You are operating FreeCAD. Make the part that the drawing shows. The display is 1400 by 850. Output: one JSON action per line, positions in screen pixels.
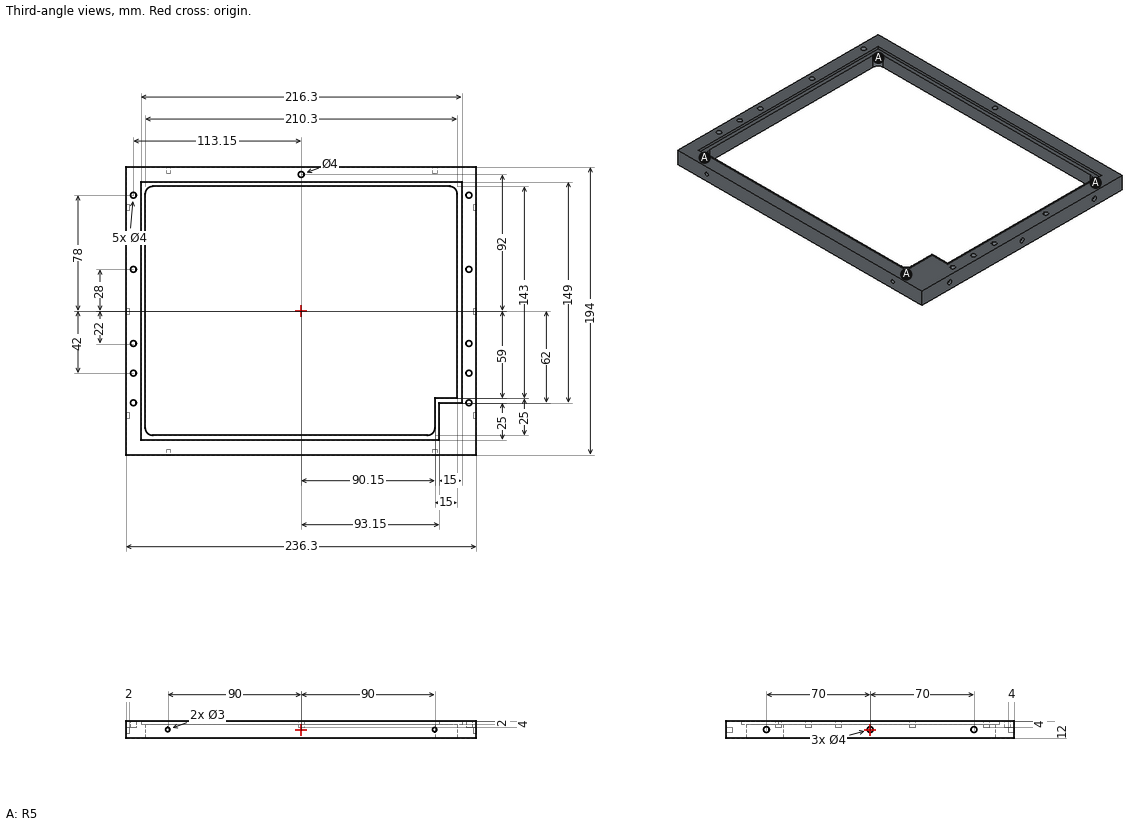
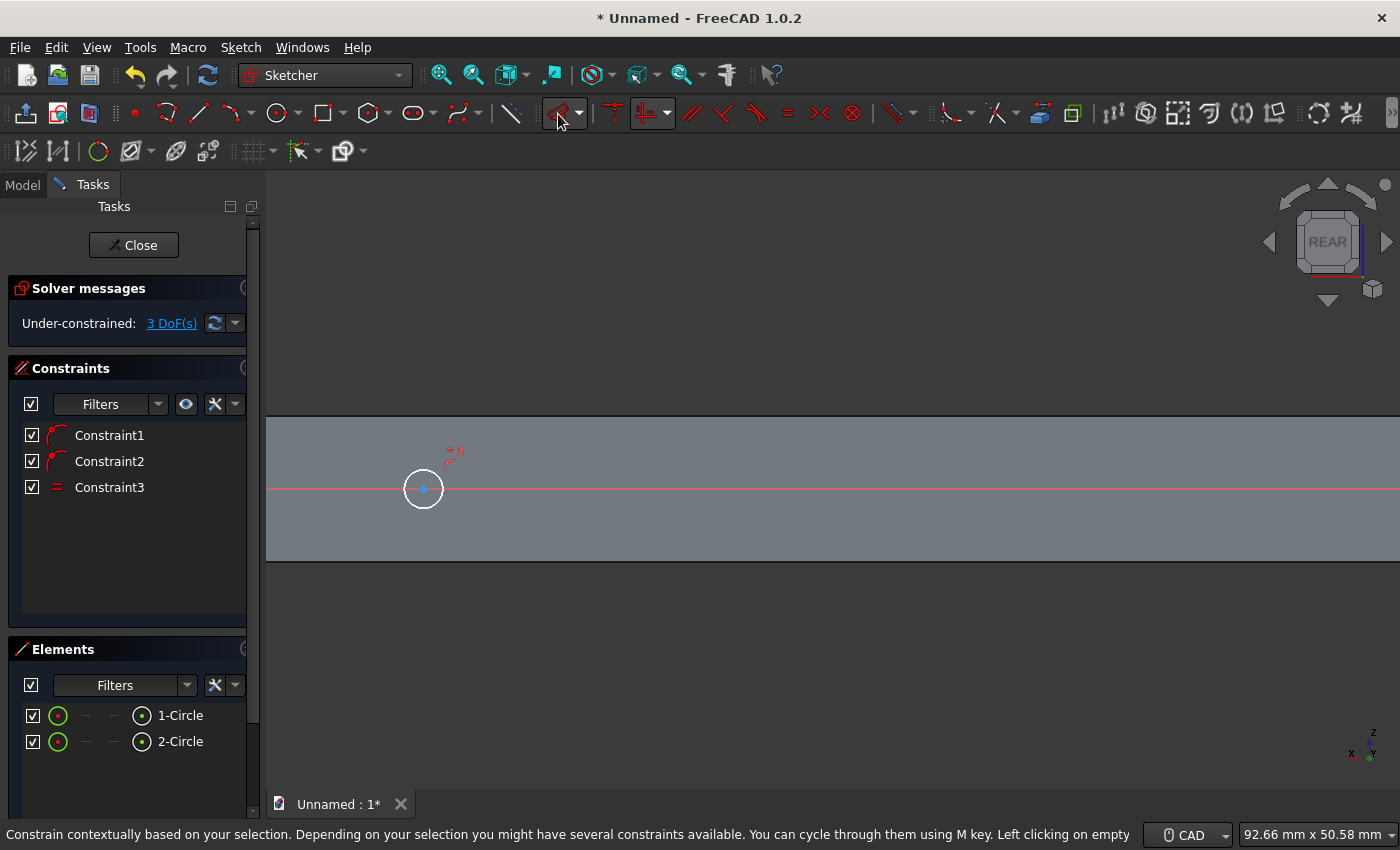
{"action": "scroll", "coordinate": [437, 475], "scroll_direction": "down", "scroll_amount": 6}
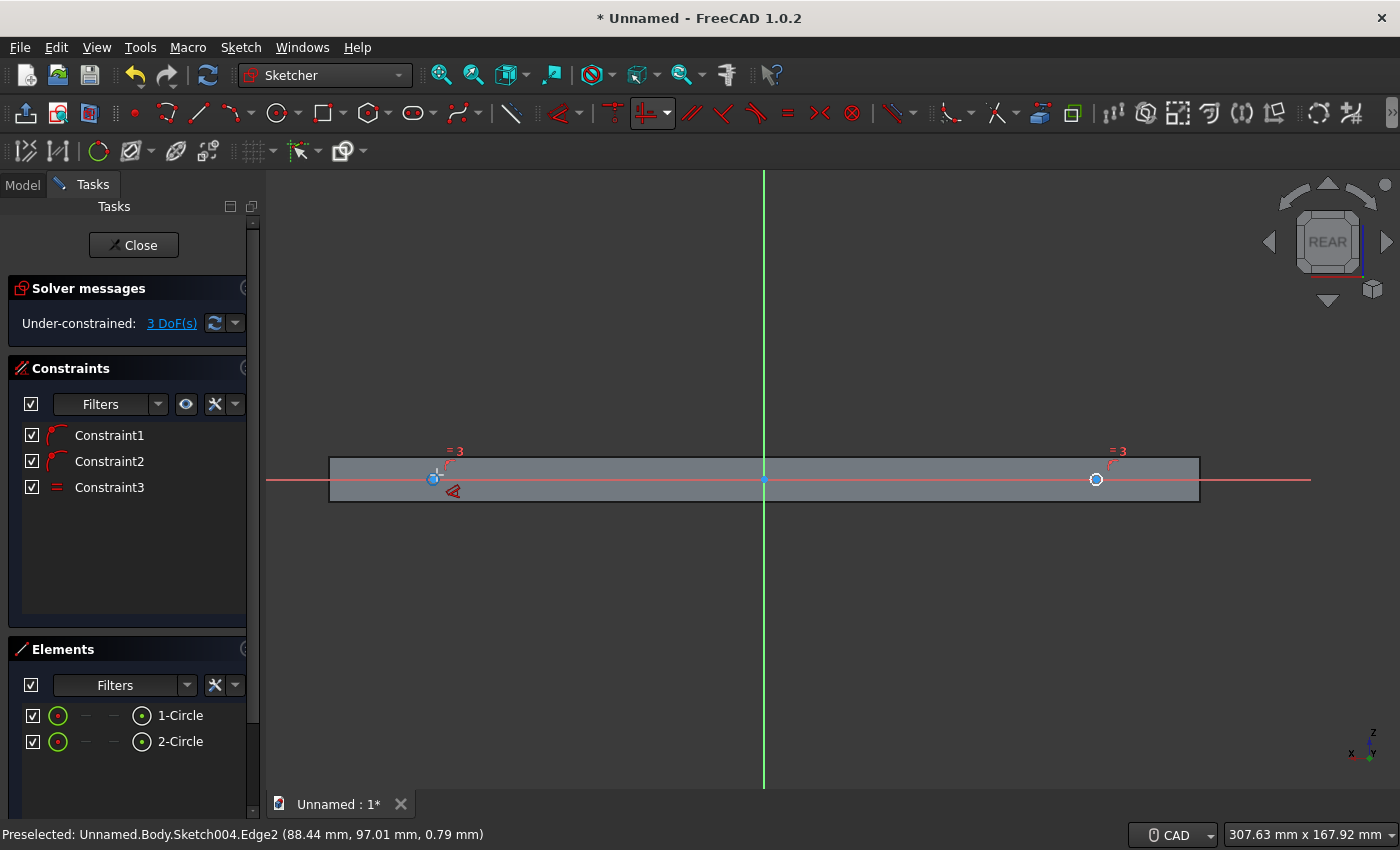
{"action": "scroll", "coordinate": [1100, 475], "scroll_direction": "up", "scroll_amount": 7}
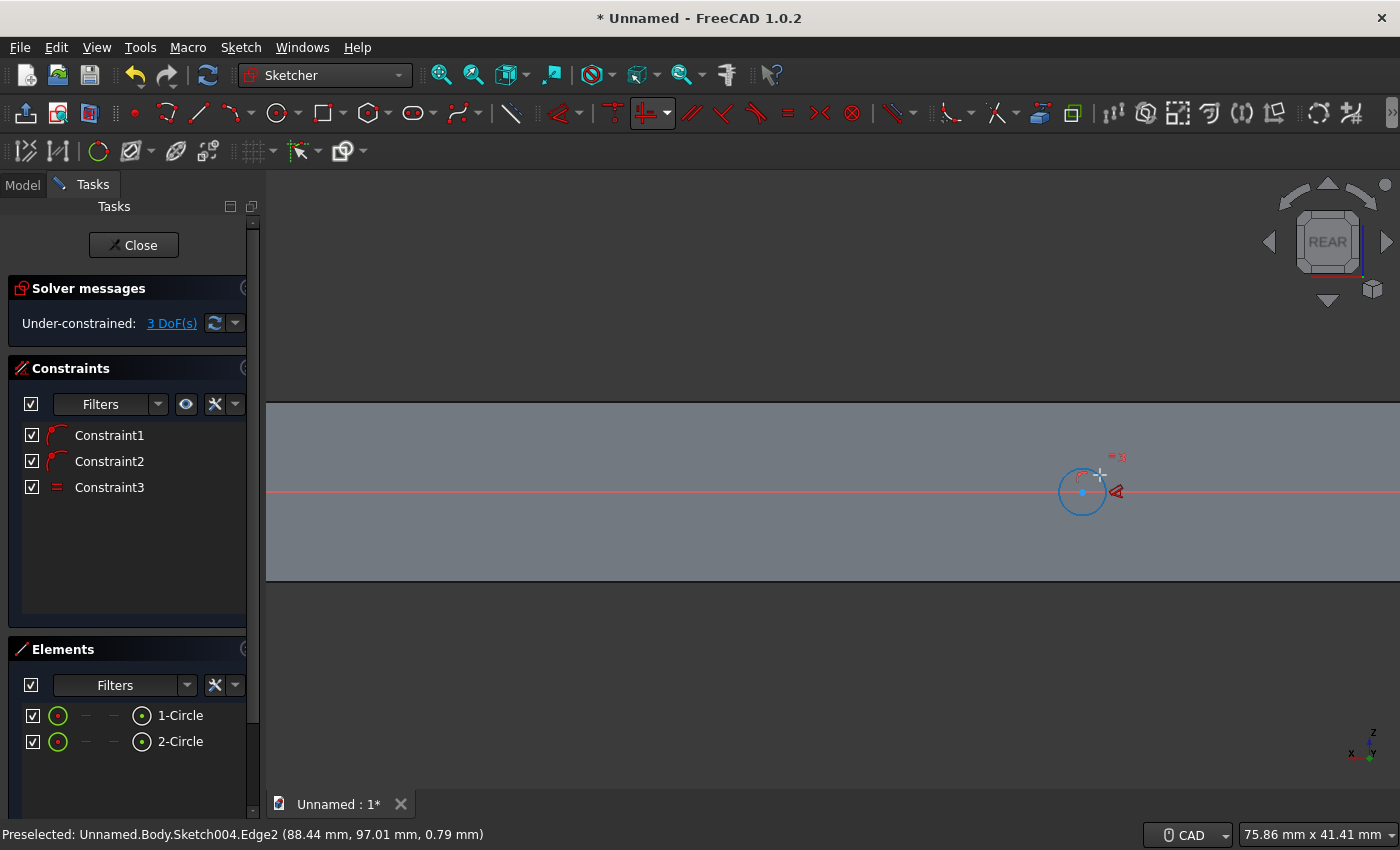
{"action": "left_click", "coordinate": [1099, 475]}
{"action": "left_click", "coordinate": [1121, 452]}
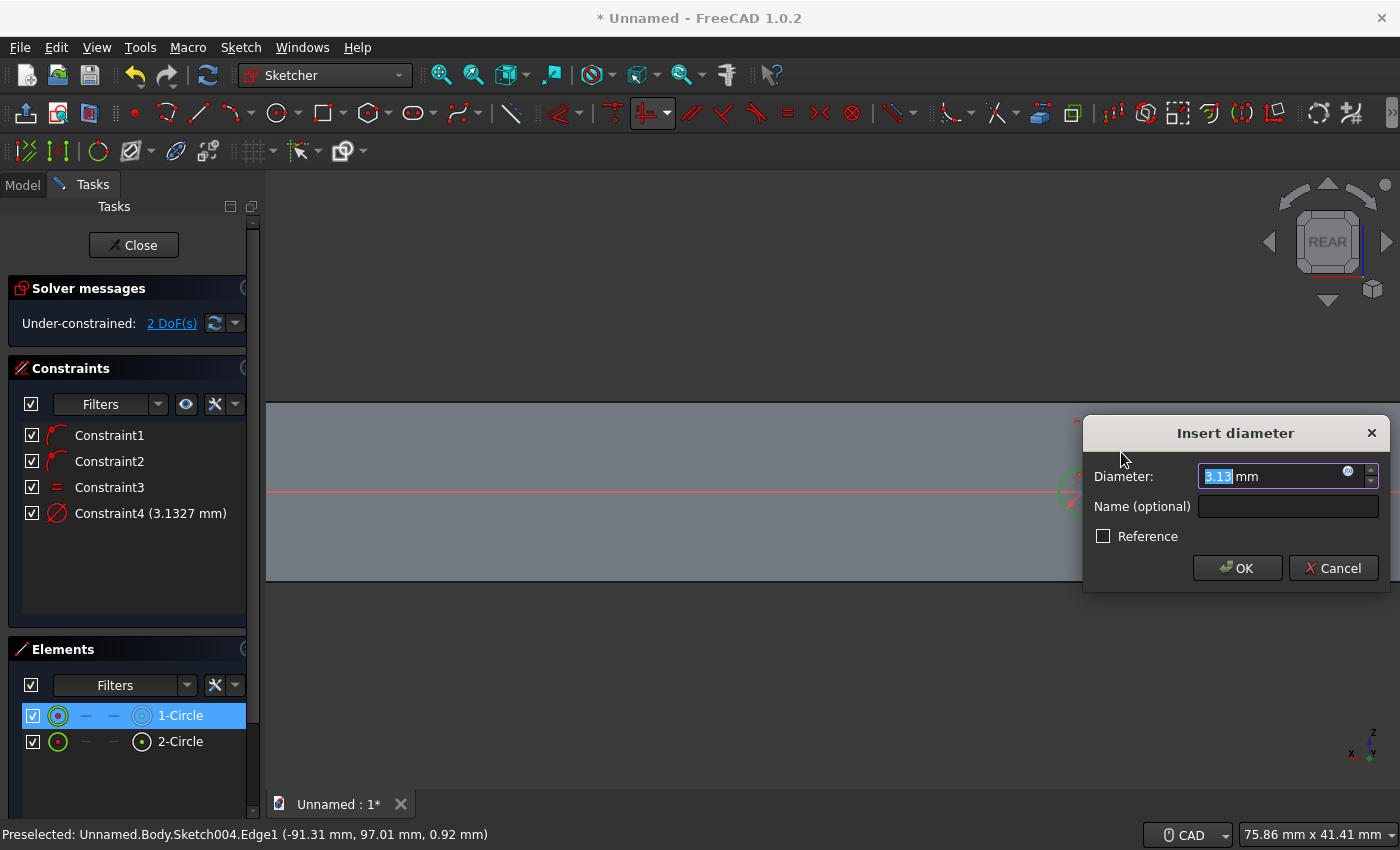
{"action": "type", "text": "3"}
{"action": "key", "text": "Return"}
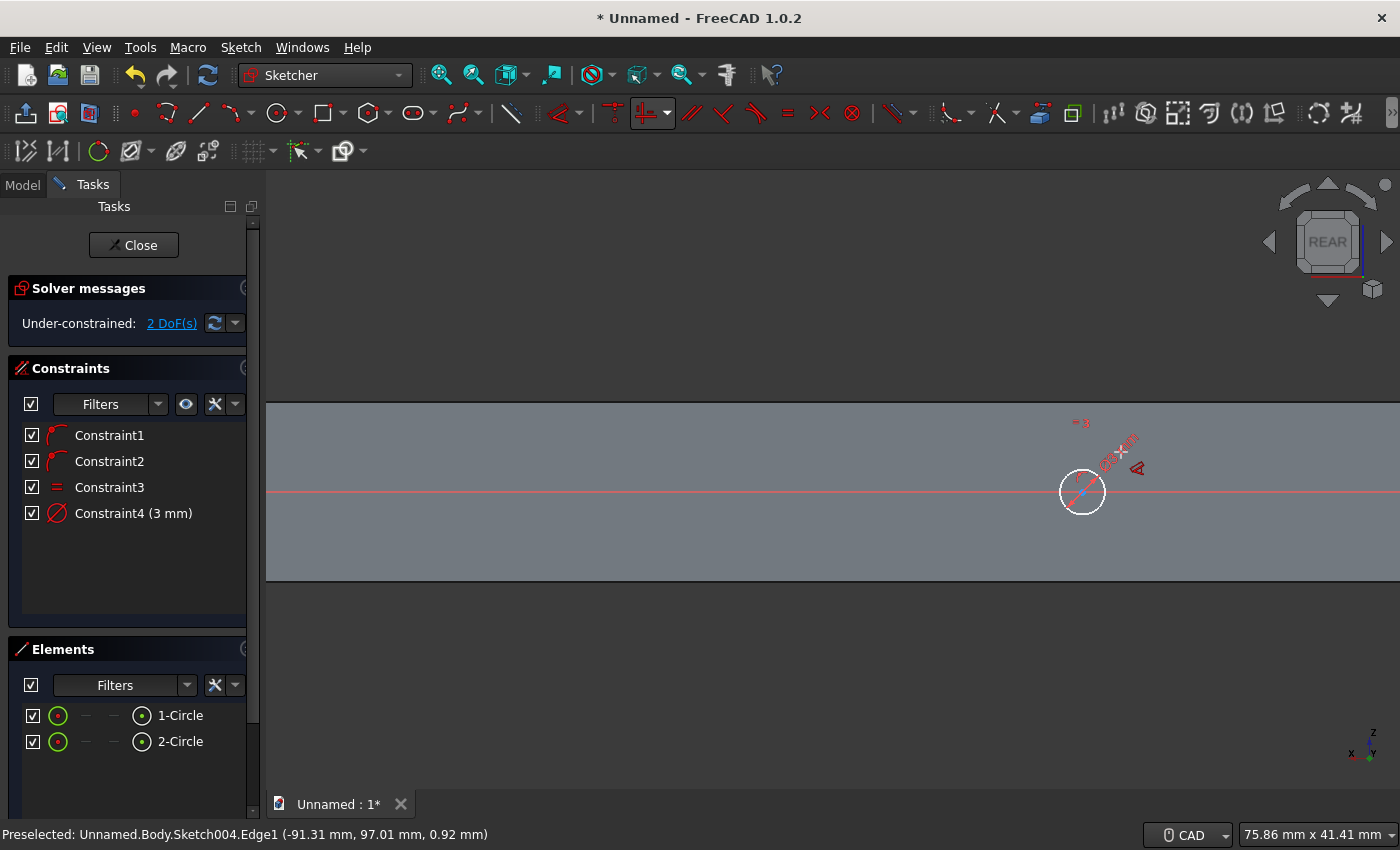
{"action": "scroll", "coordinate": [1101, 475], "scroll_direction": "down", "scroll_amount": 7}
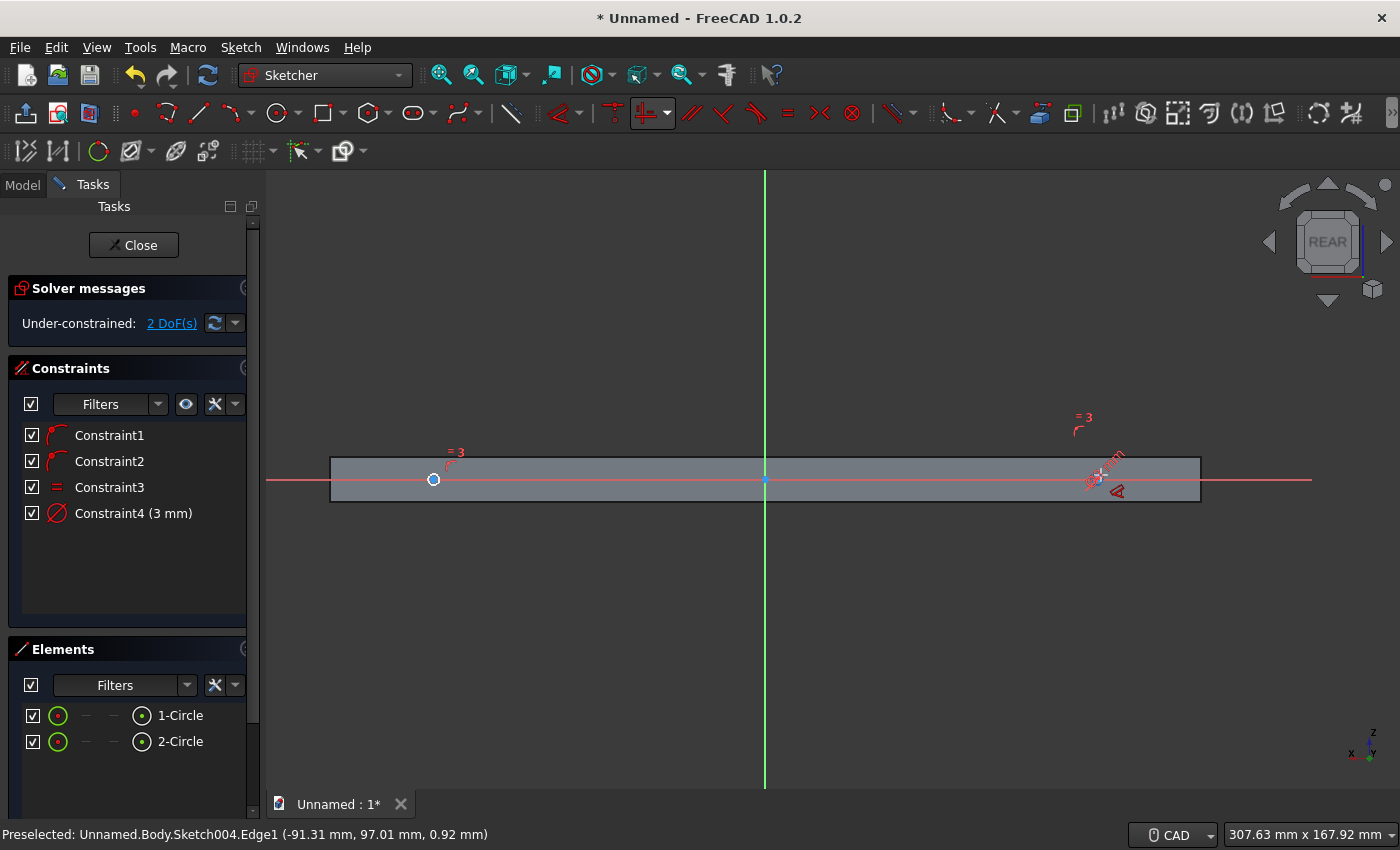
{"action": "left_click", "coordinate": [1097, 480]}
{"action": "left_click", "coordinate": [931, 514]}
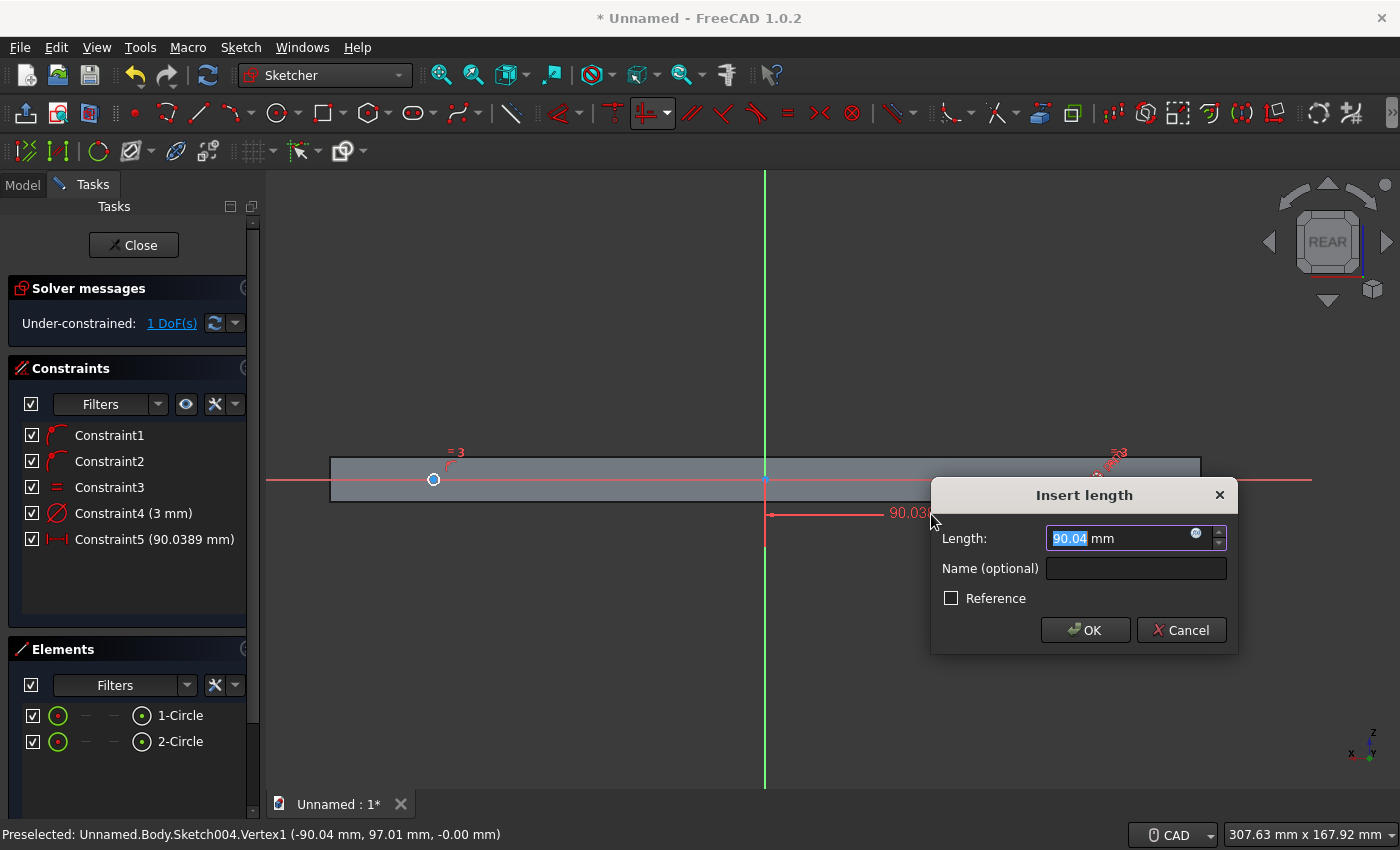
{"action": "type", "text": "90"}
{"action": "key", "text": "Return"}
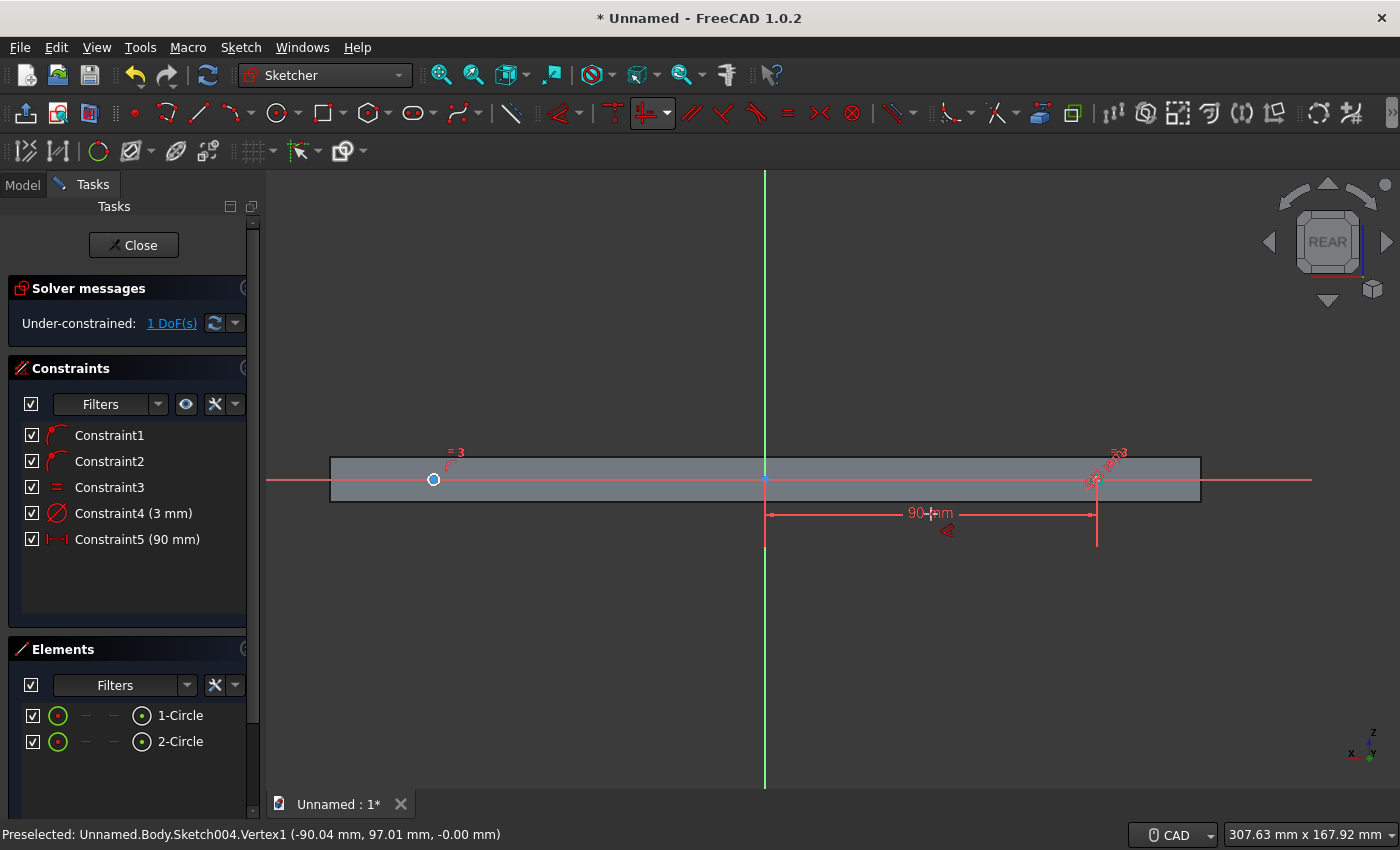
{"action": "left_click", "coordinate": [434, 480]}
{"action": "left_click", "coordinate": [599, 514]}